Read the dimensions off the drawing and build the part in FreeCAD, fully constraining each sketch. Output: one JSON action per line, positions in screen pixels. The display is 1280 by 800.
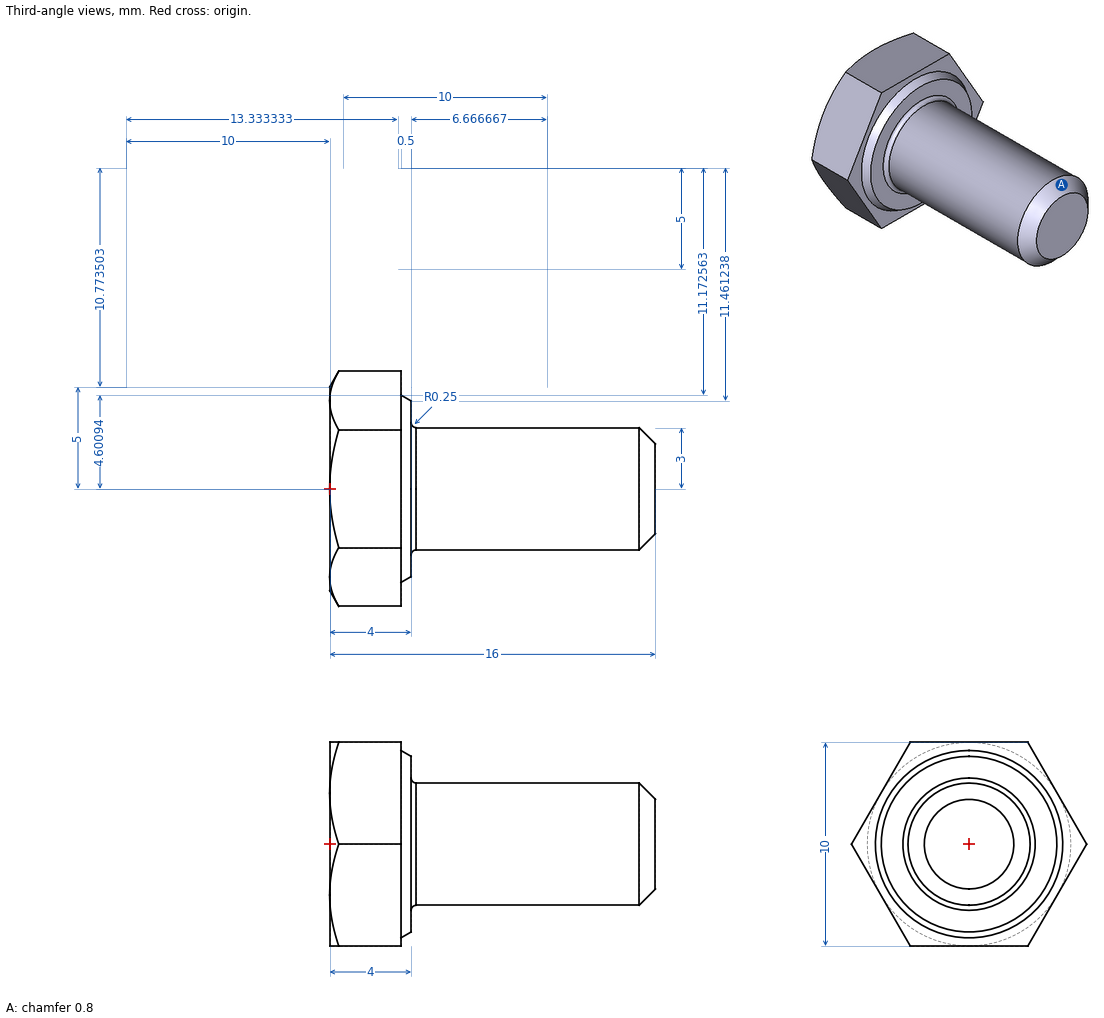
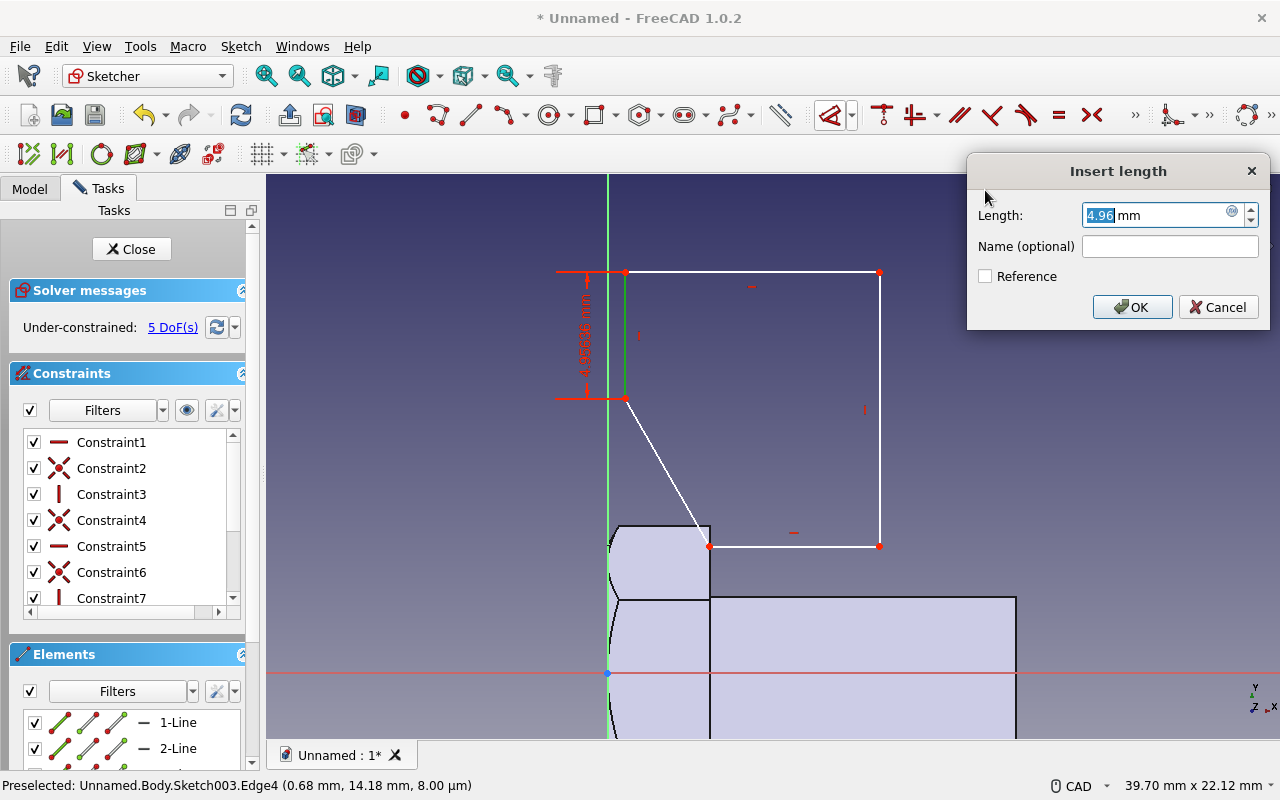
{"action": "type", "text": "5"}
{"action": "key", "text": "Return"}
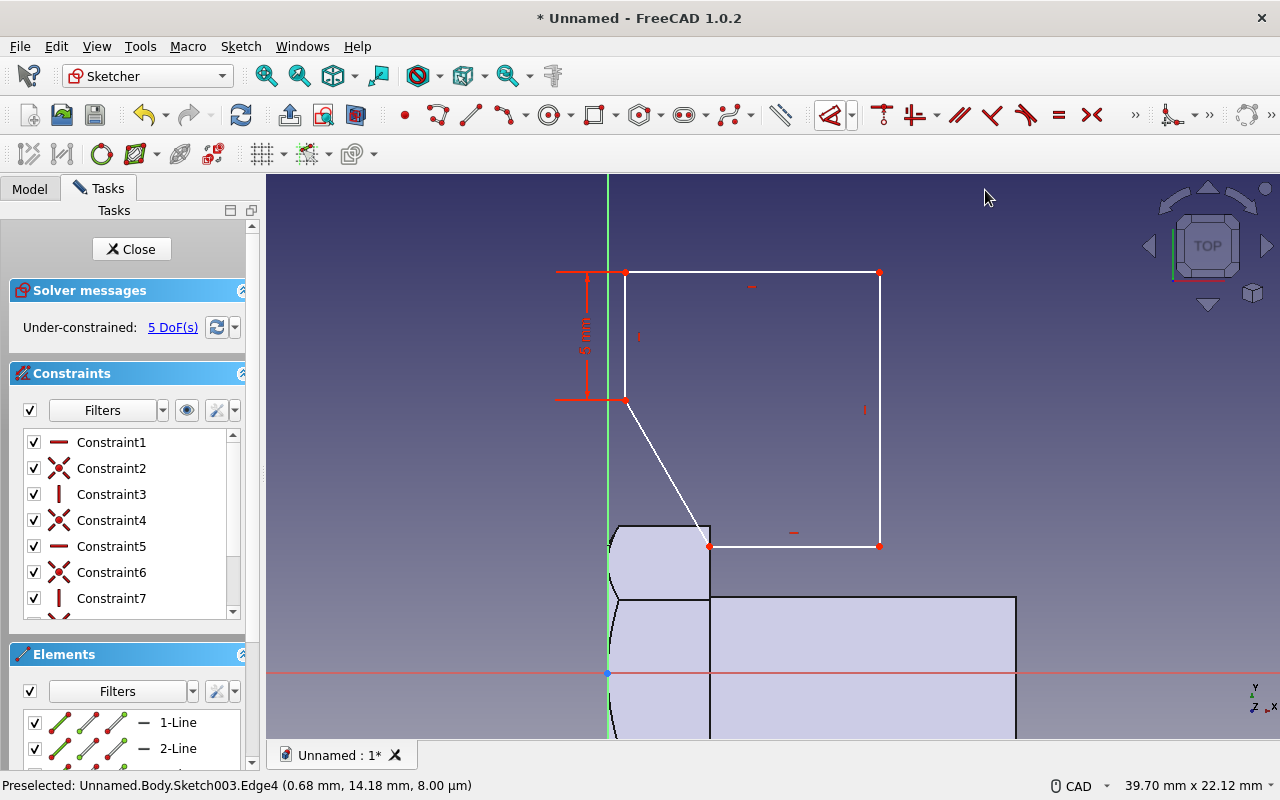
{"action": "left_click", "coordinate": [803, 272]}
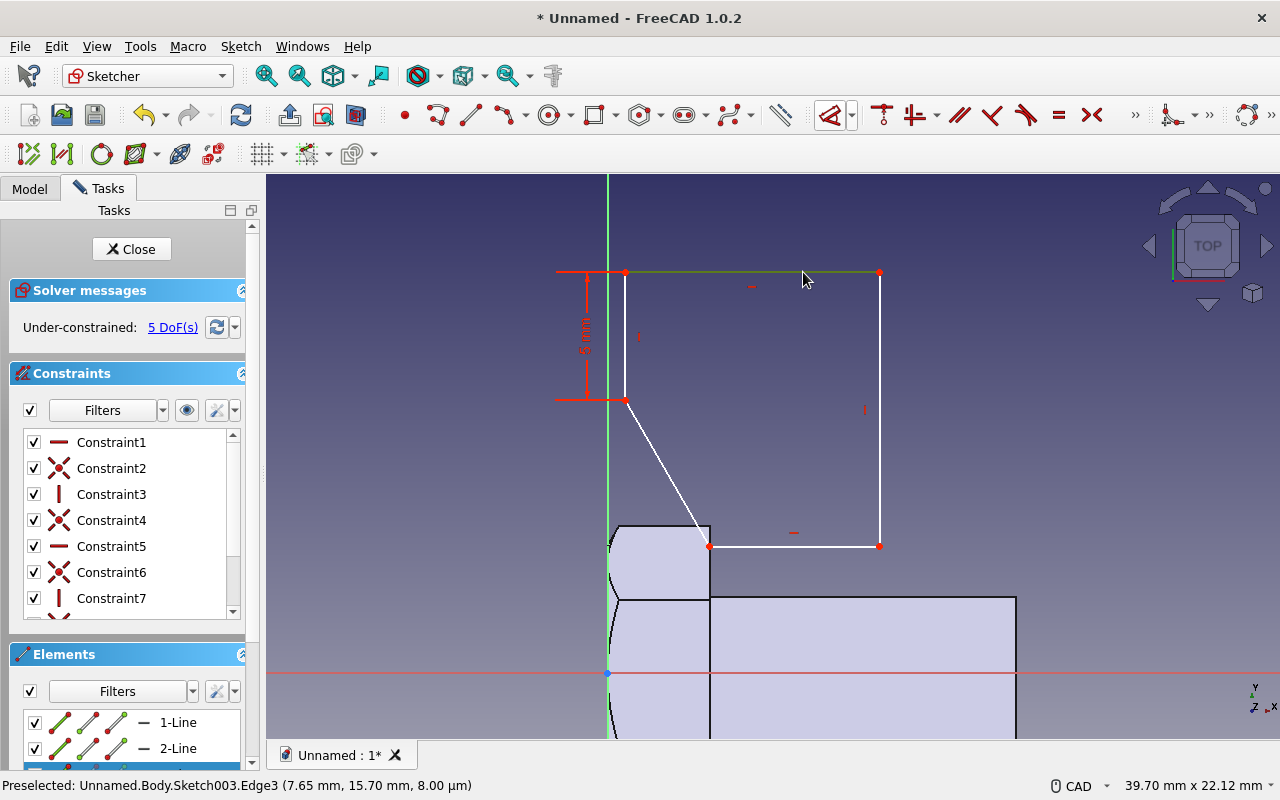
{"action": "left_click", "coordinate": [852, 116]}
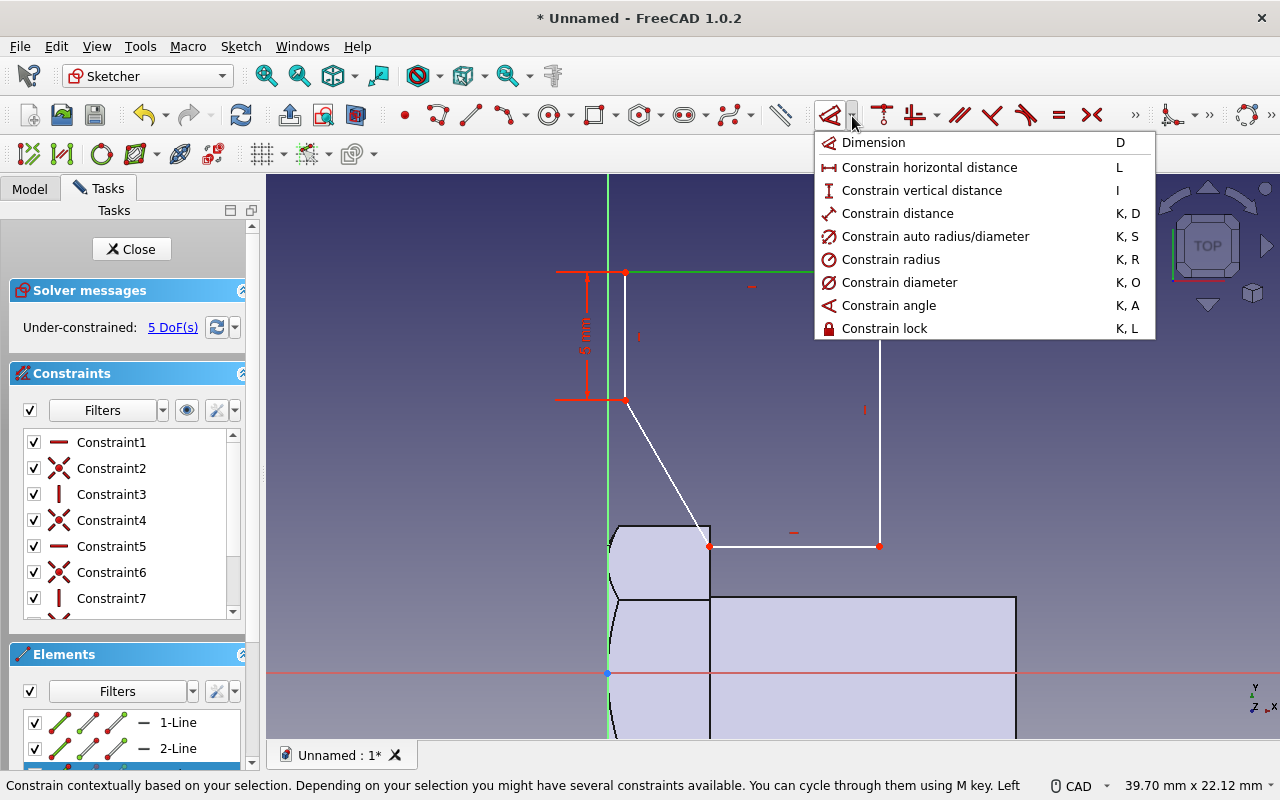
{"action": "left_click", "coordinate": [985, 168]}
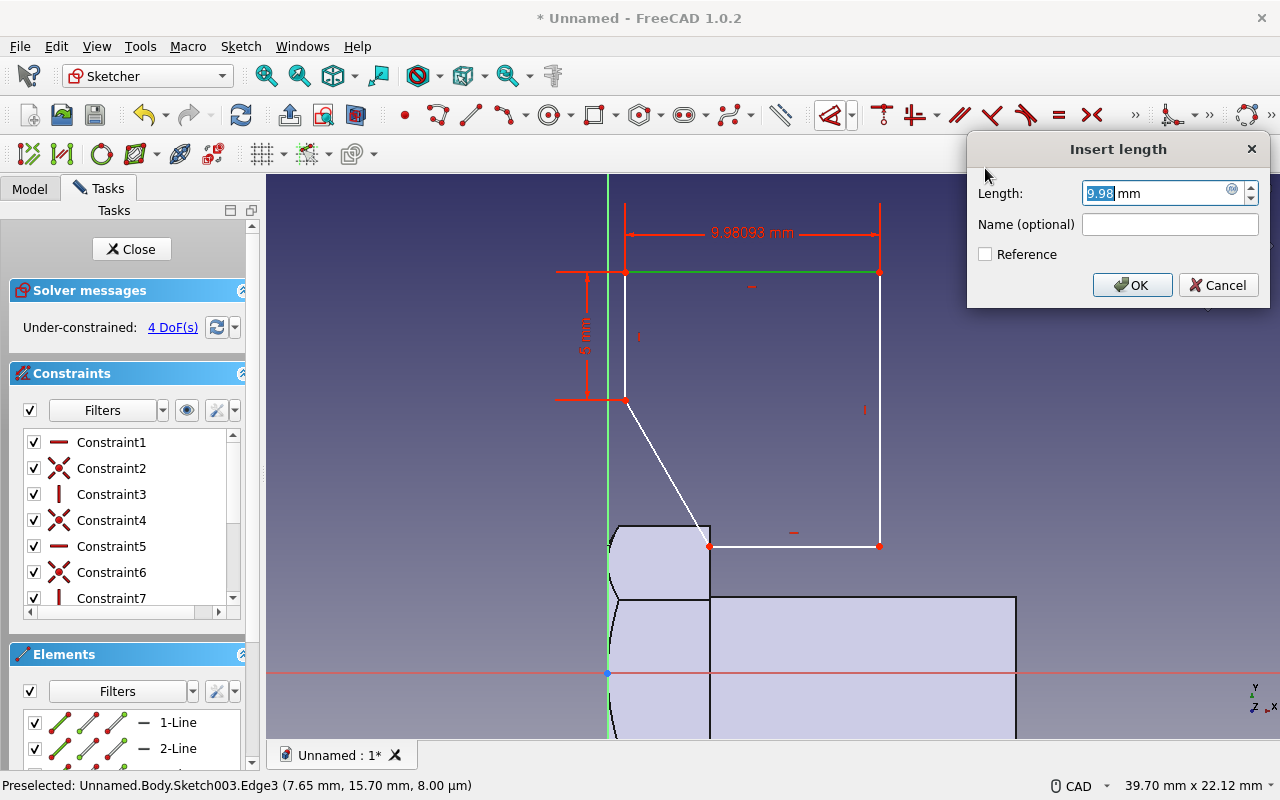
{"action": "type", "text": "10"}
{"action": "key", "text": "Return"}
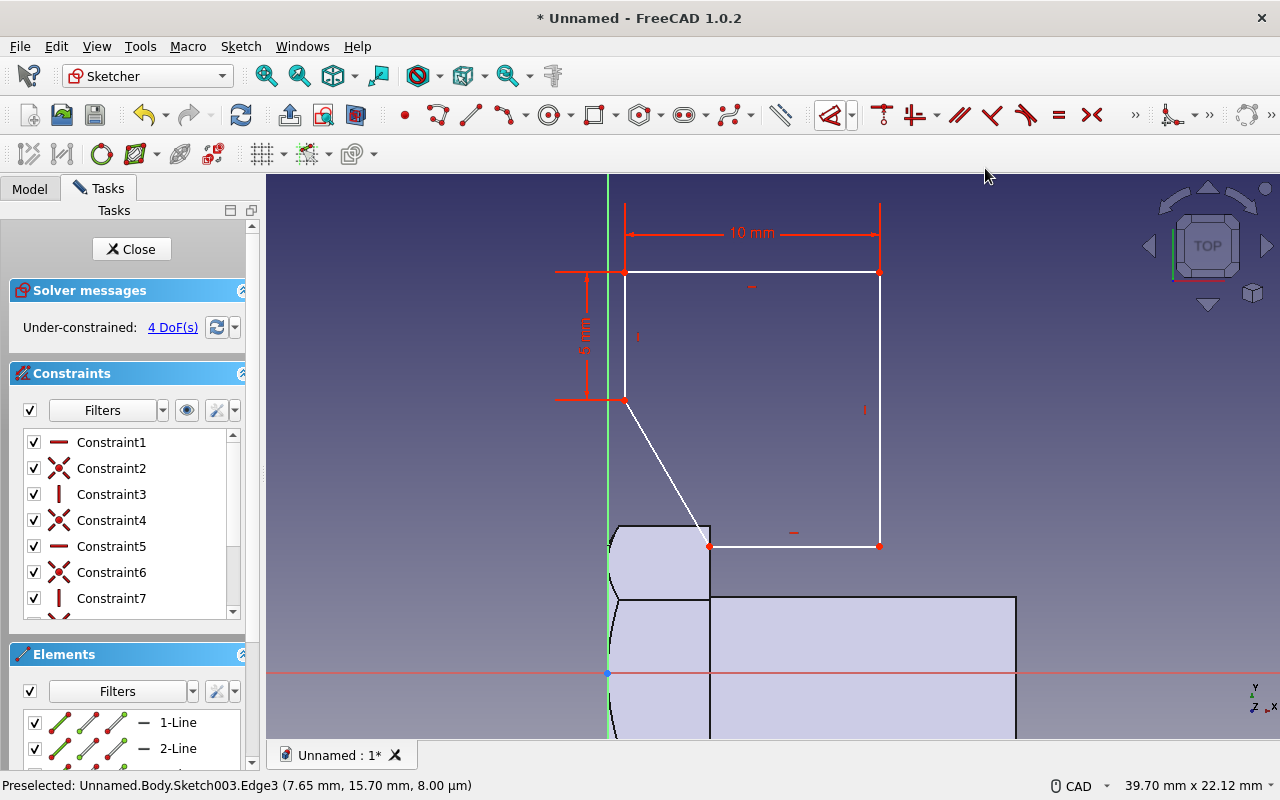
{"action": "left_click", "coordinate": [710, 547]}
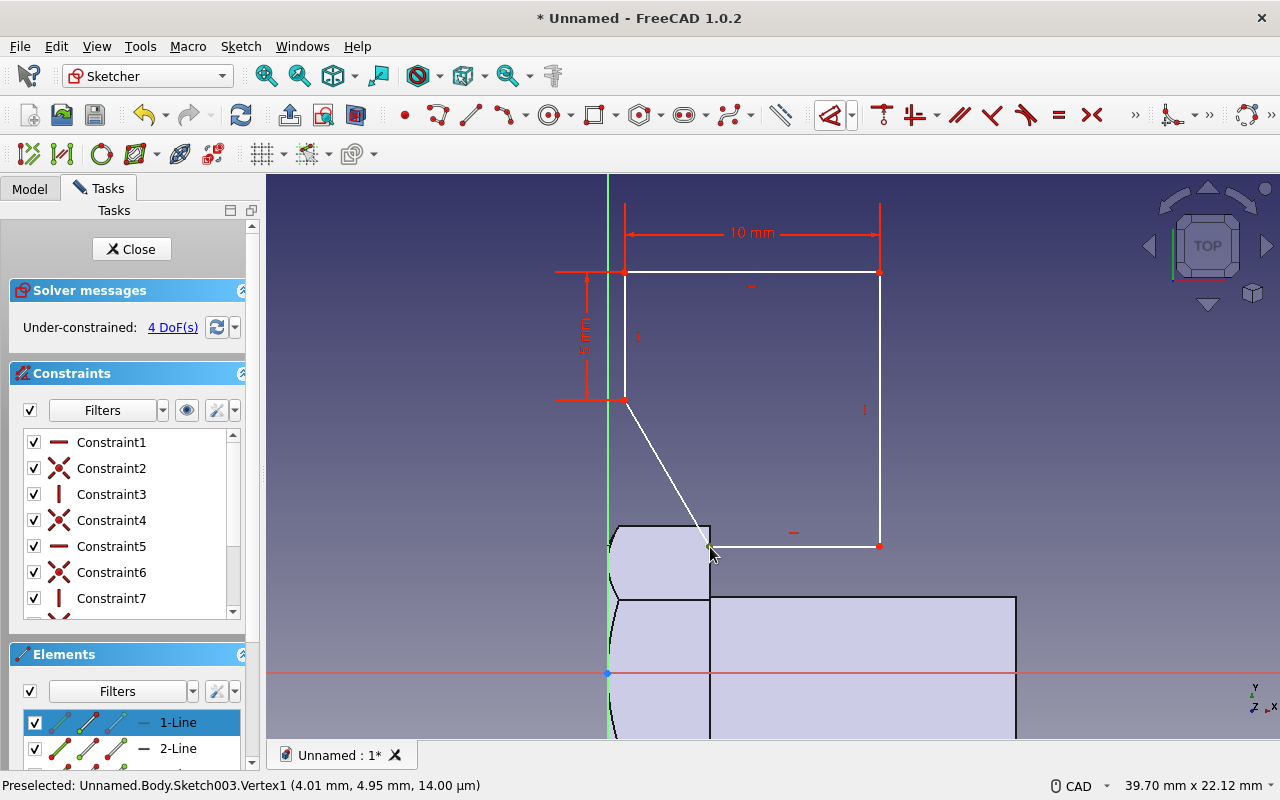
{"action": "left_click", "coordinate": [852, 116]}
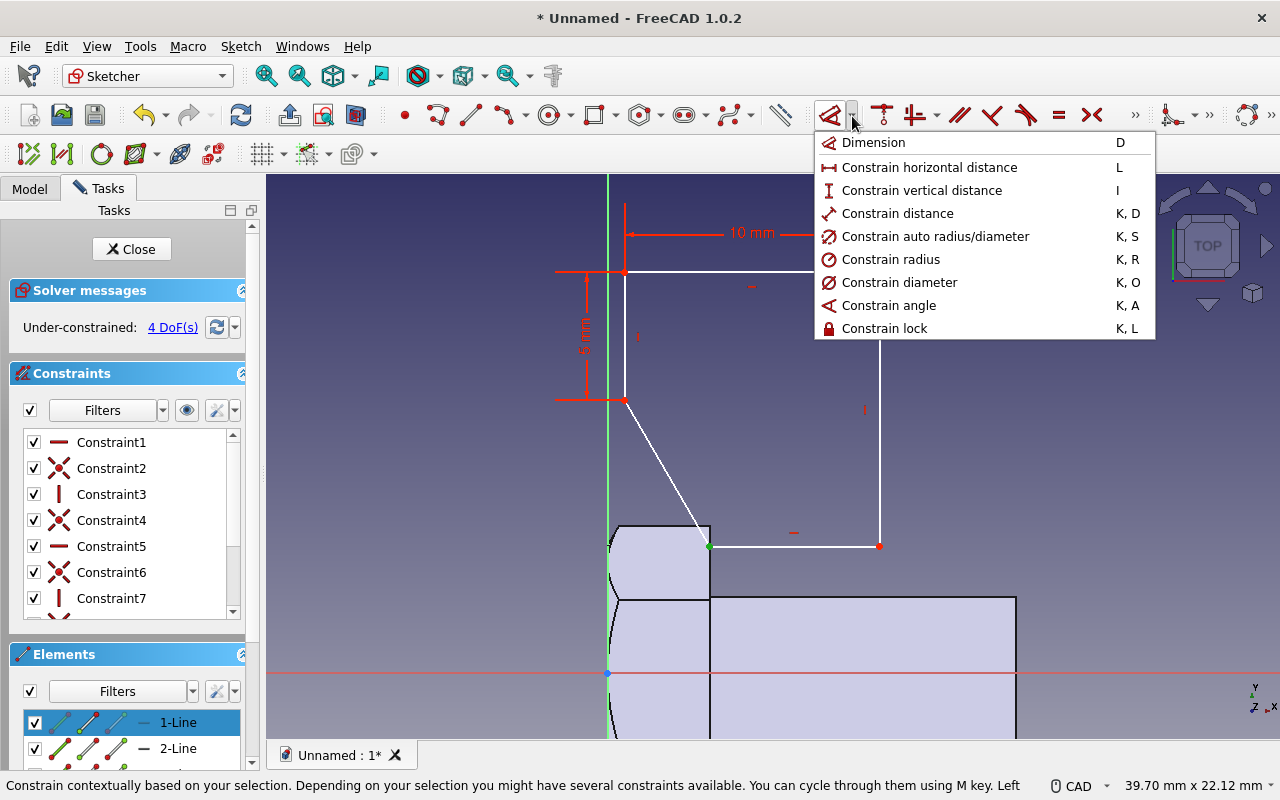
{"action": "left_click", "coordinate": [985, 168]}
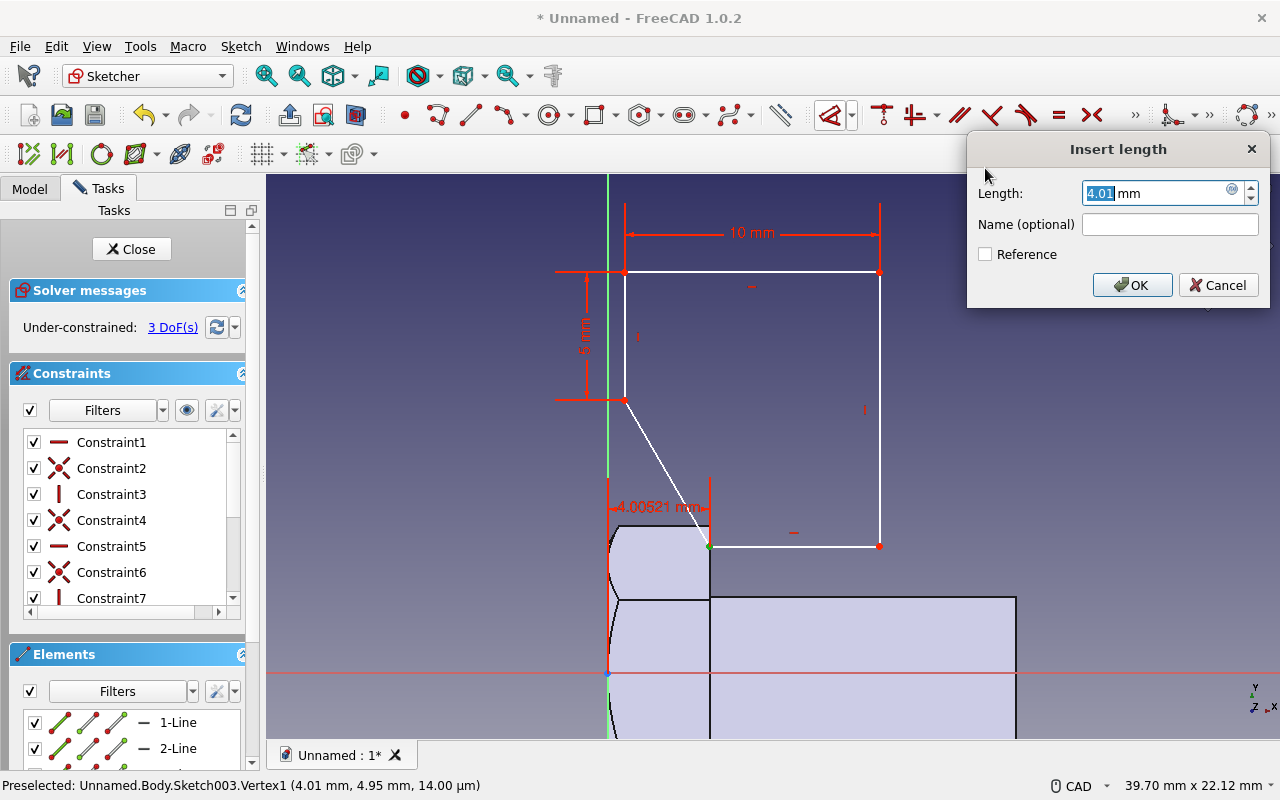
{"action": "type", "text": "4"}
{"action": "key", "text": "Return"}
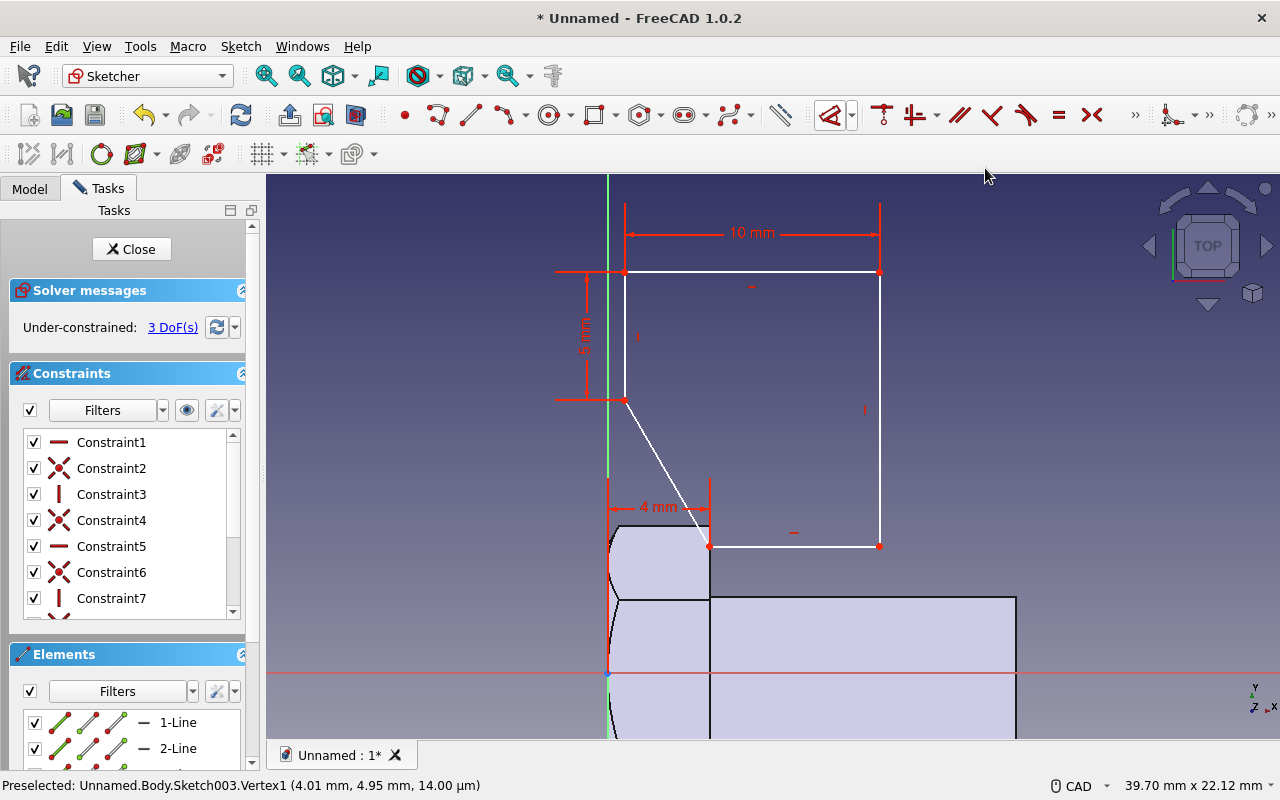
{"action": "left_click", "coordinate": [710, 547]}